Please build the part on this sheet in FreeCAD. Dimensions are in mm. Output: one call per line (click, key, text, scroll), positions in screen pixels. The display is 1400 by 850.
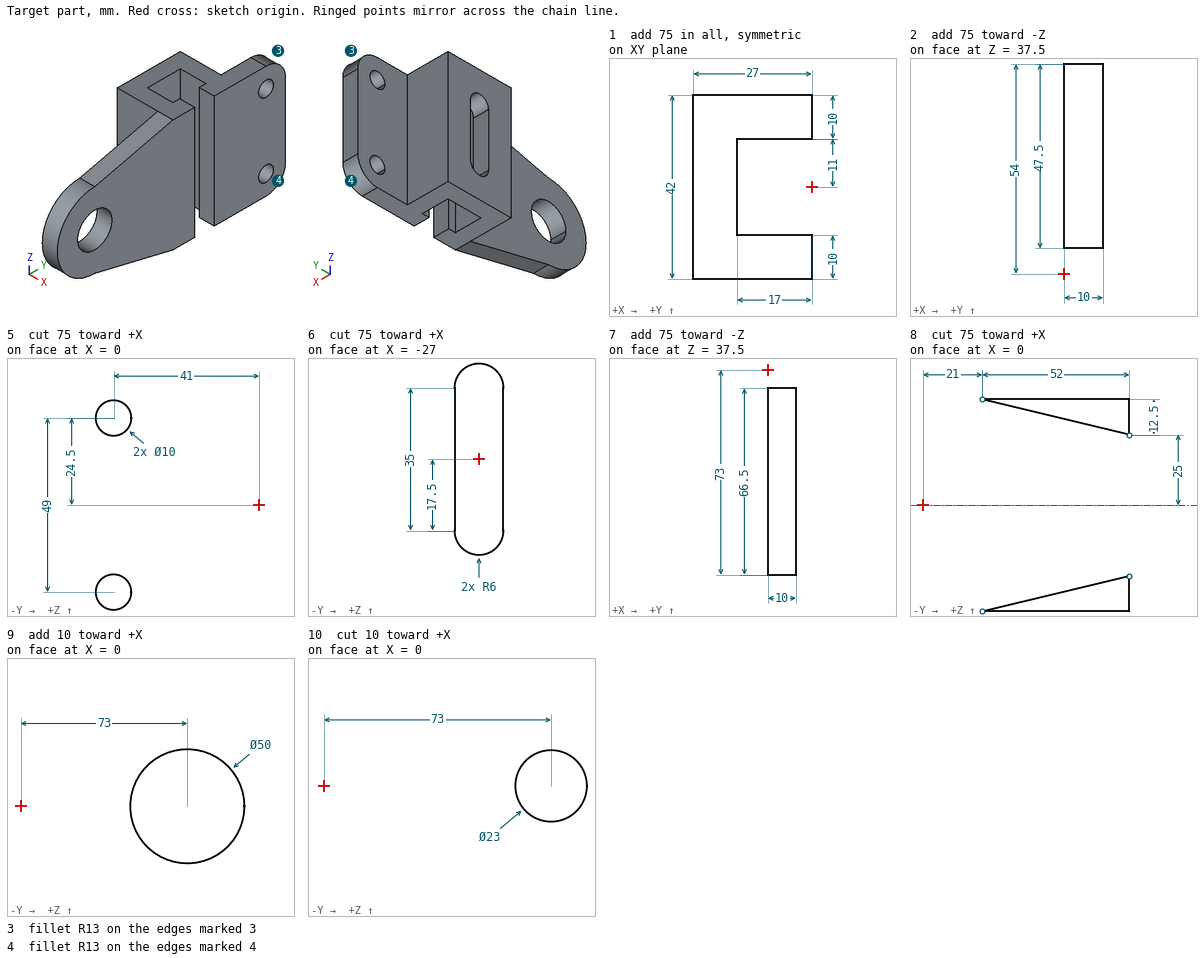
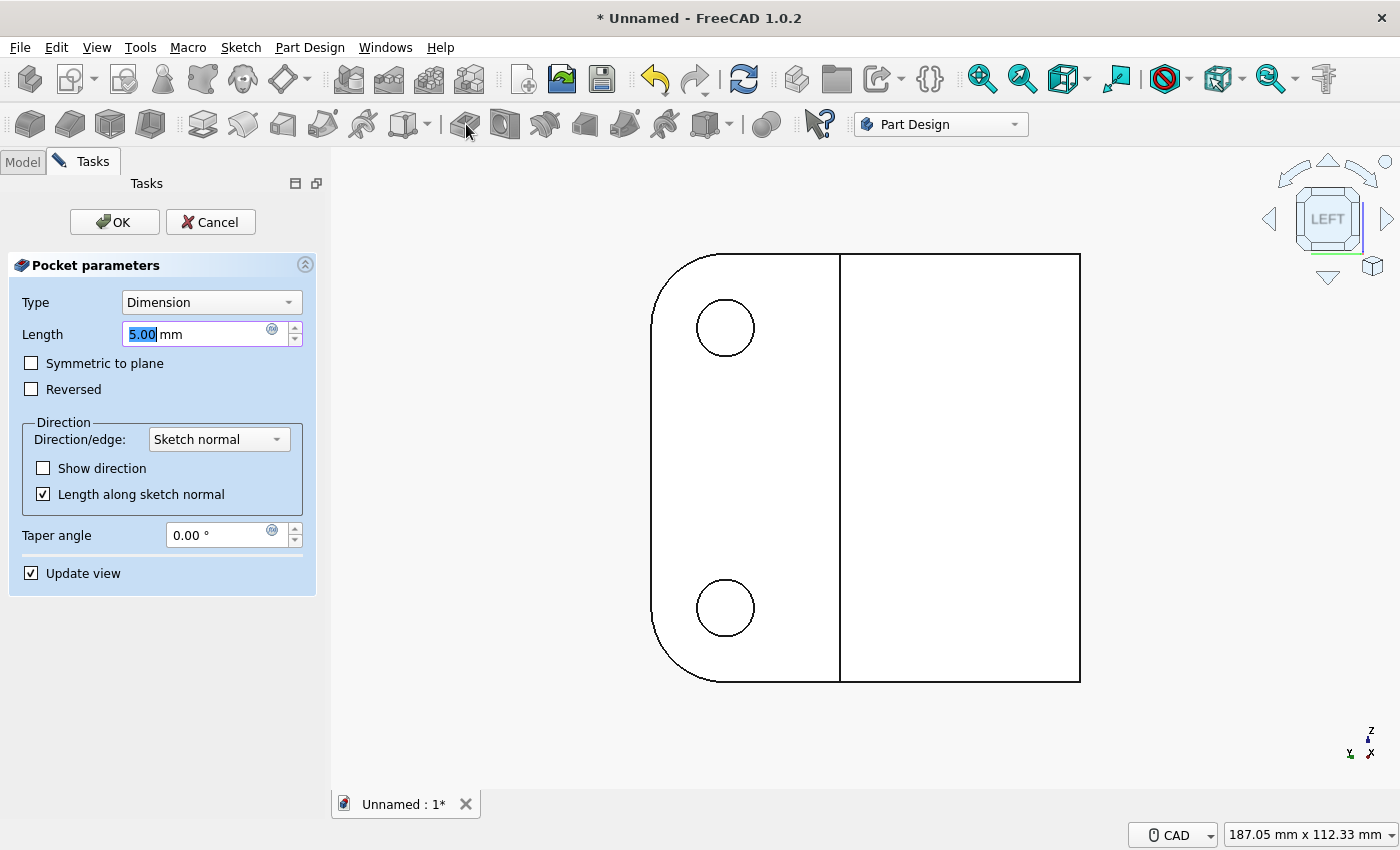
text(75)
key(Tab)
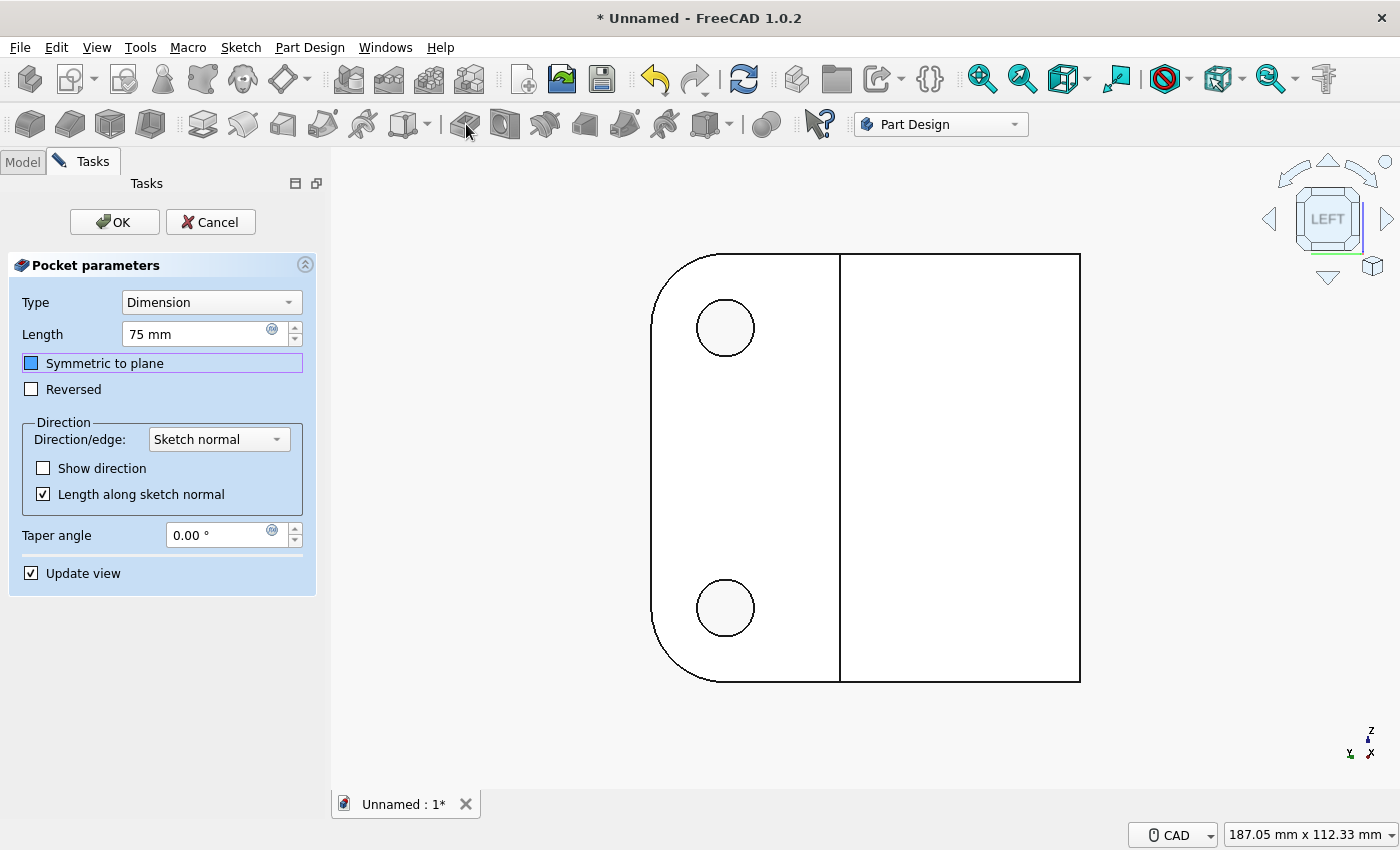
click(115, 222)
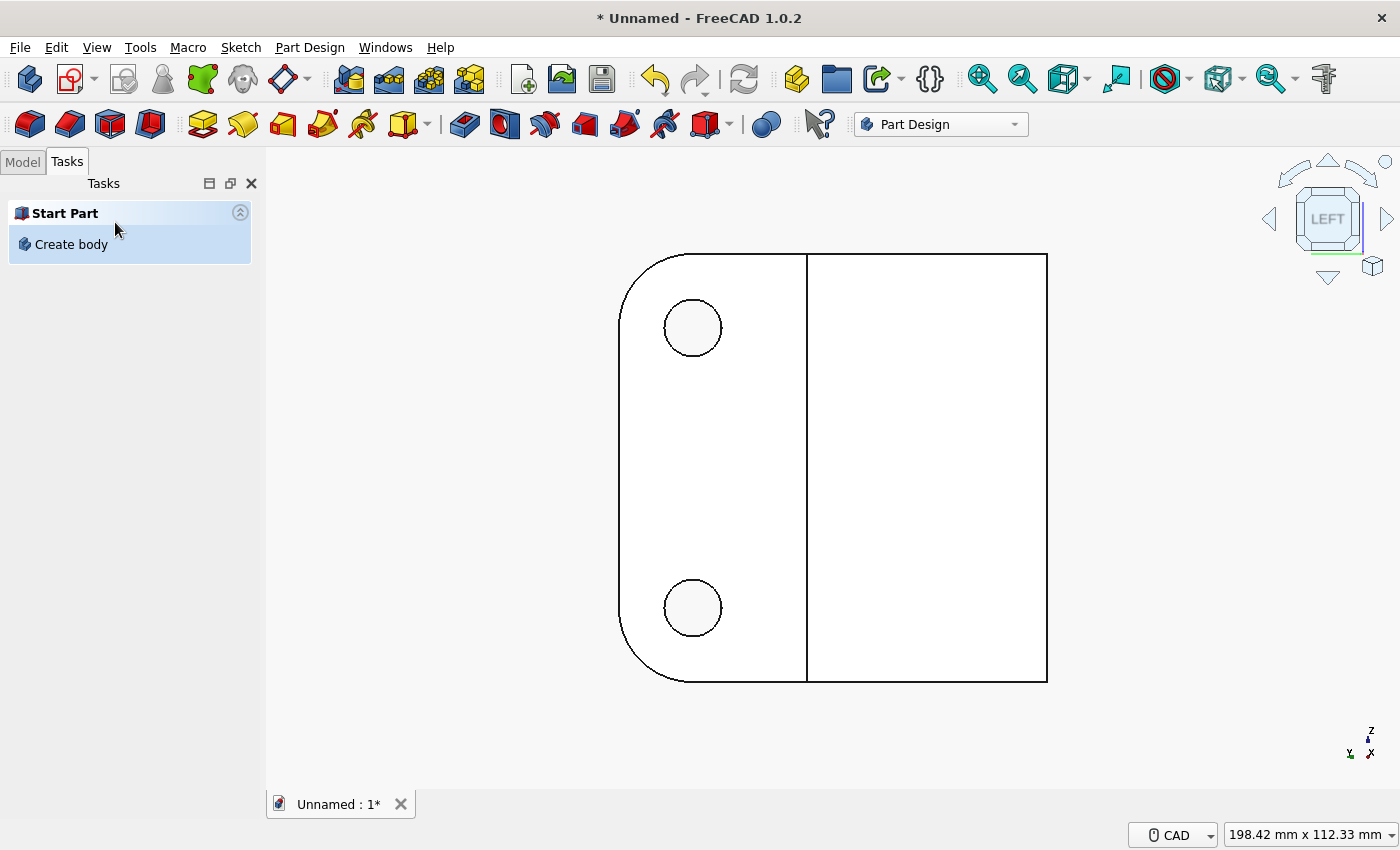
click(927, 406)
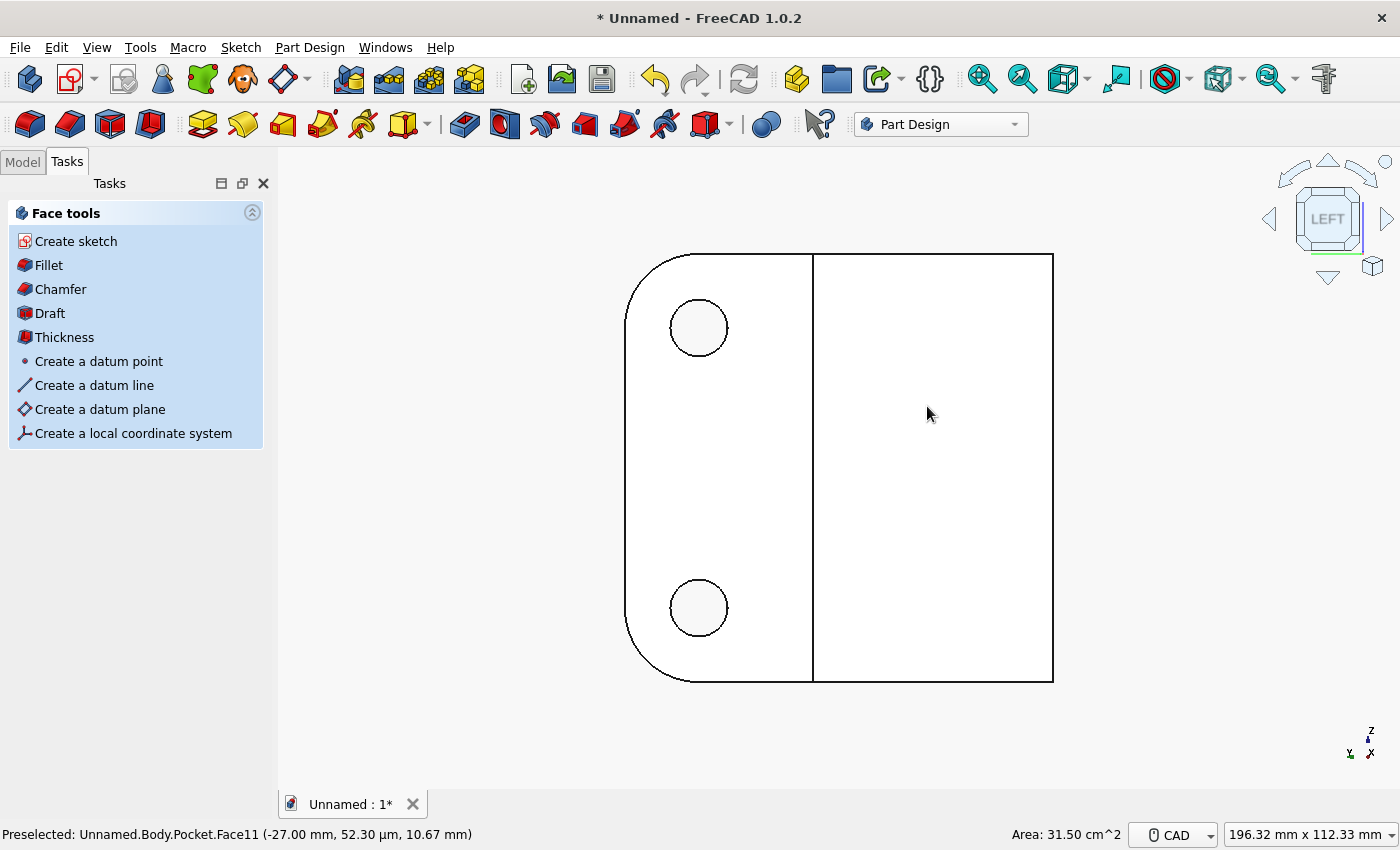
click(70, 80)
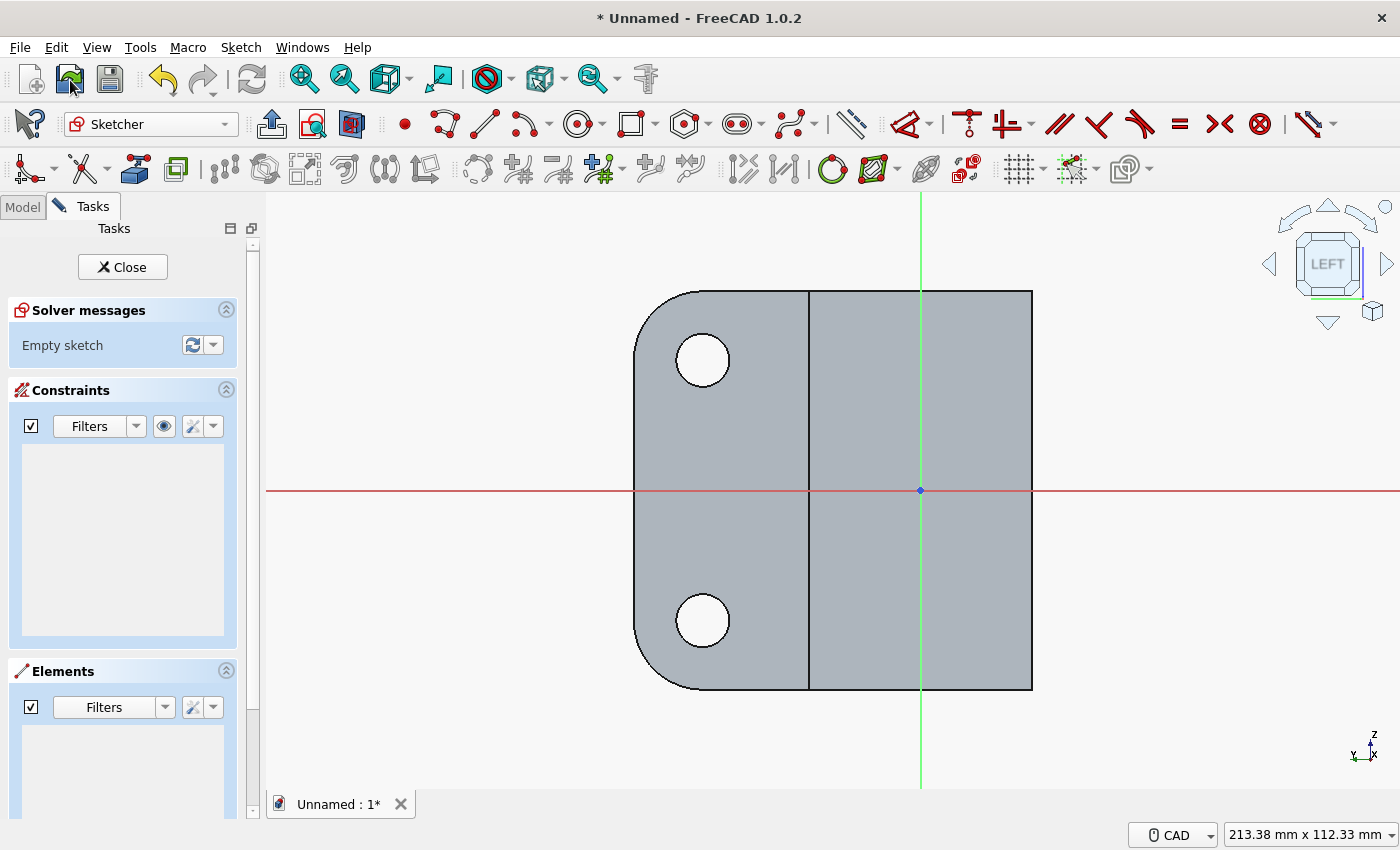
scroll(1235, 491, up, 2)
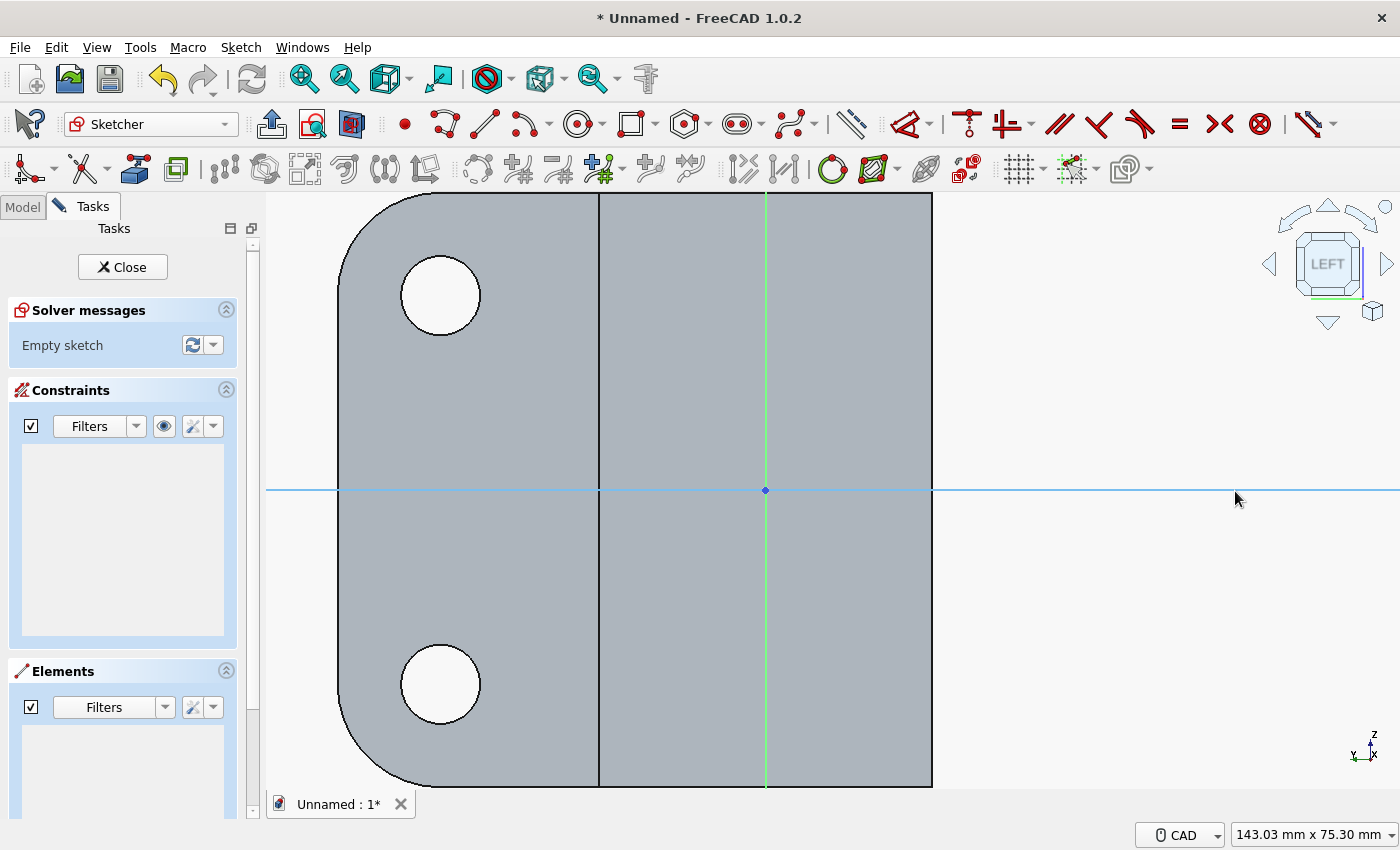
key(g)
key(s)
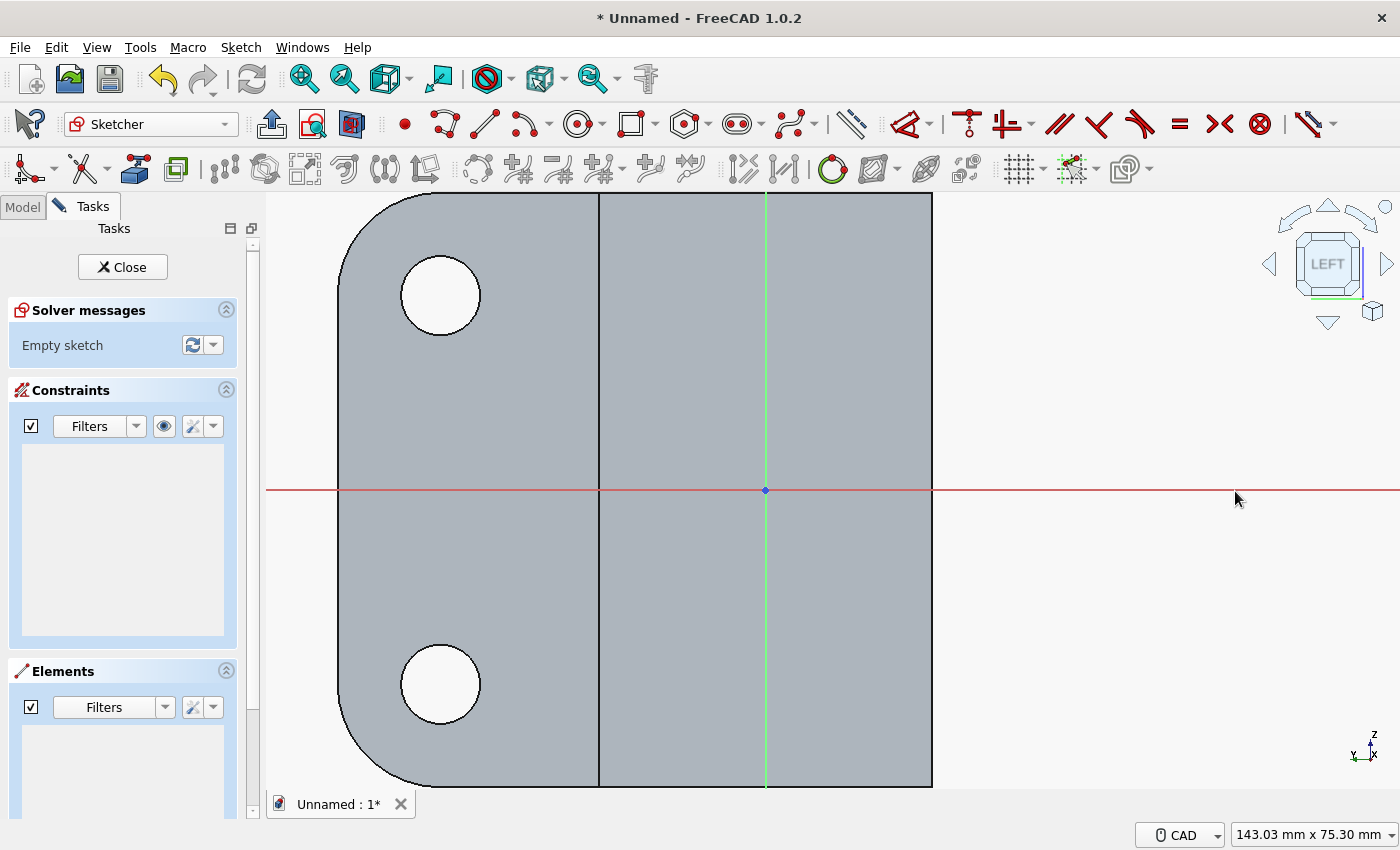
click(766, 629)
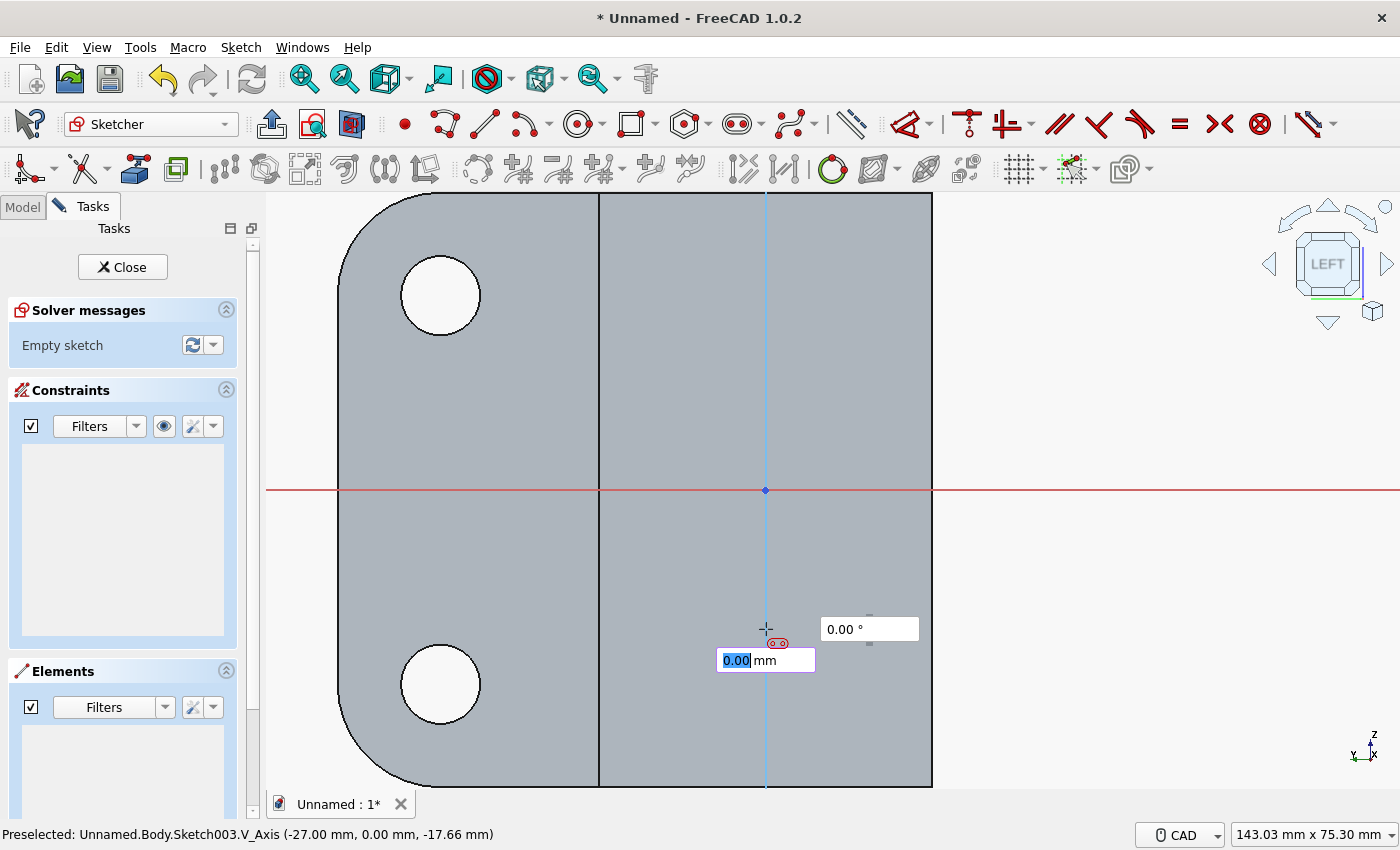
click(775, 351)